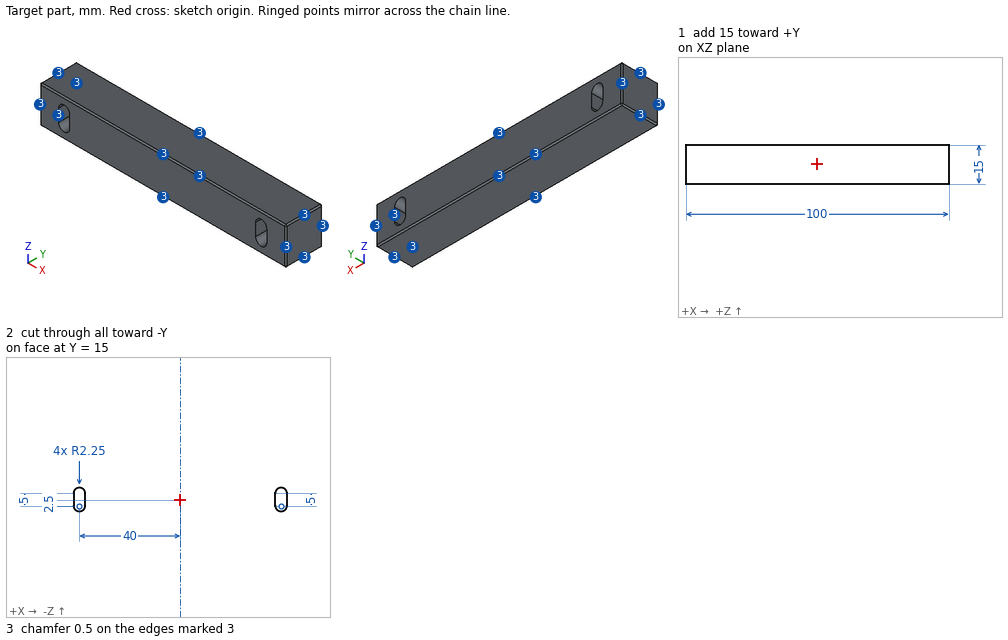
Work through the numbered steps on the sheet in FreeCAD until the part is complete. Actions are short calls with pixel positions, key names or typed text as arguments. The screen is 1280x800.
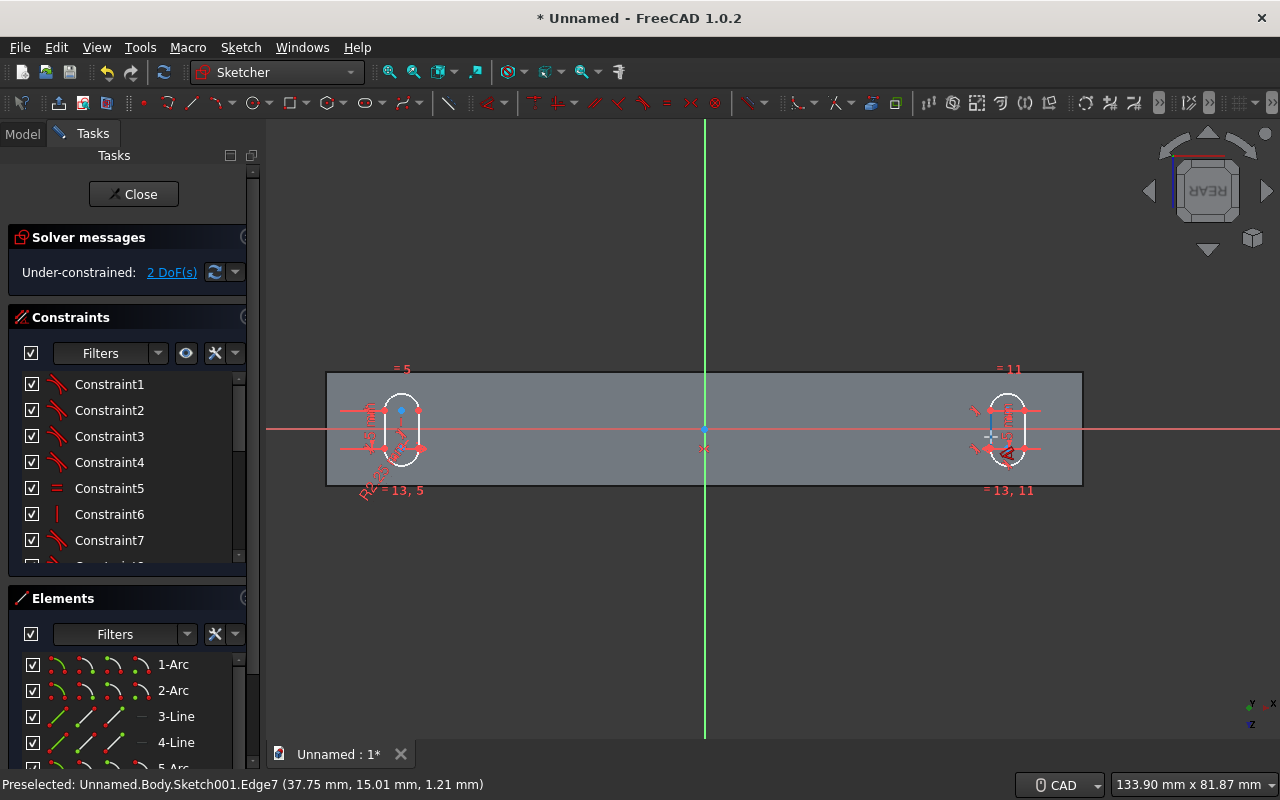
click(402, 449)
click(553, 483)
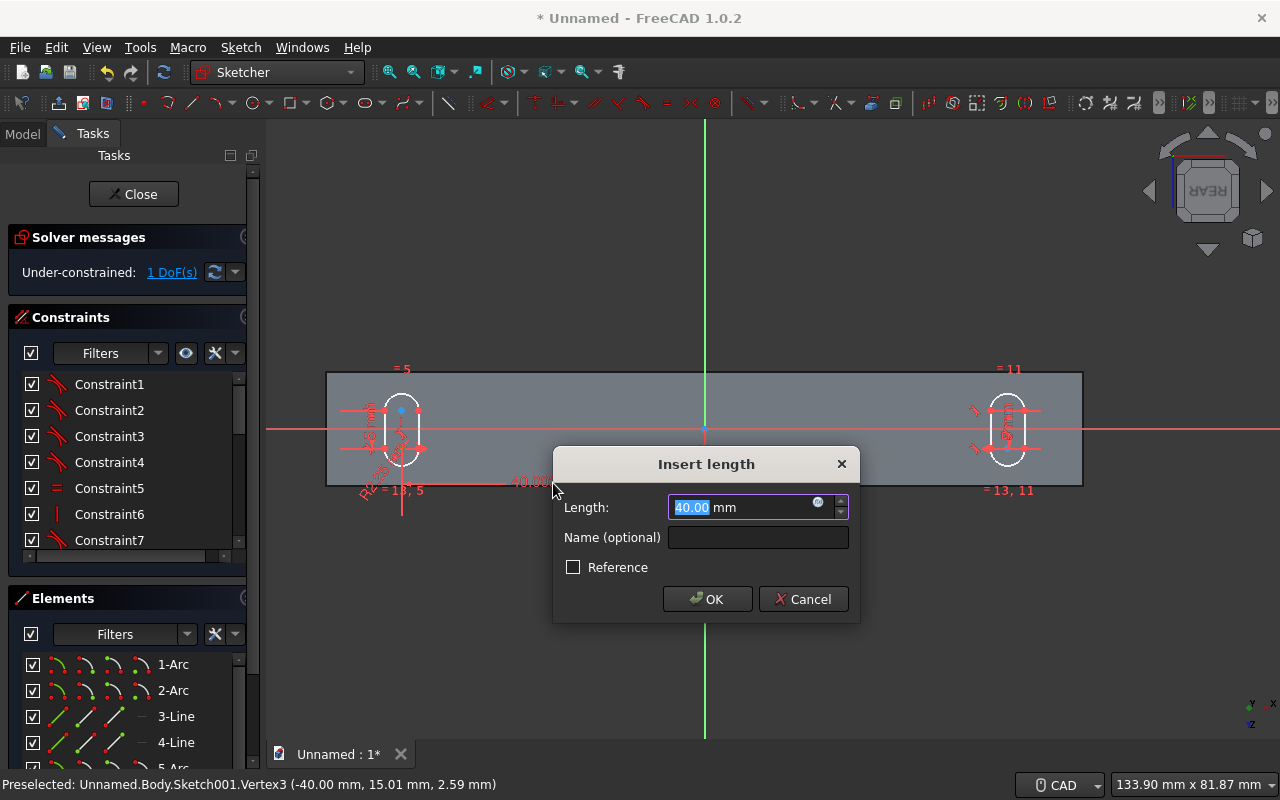
text(40)
key(Return)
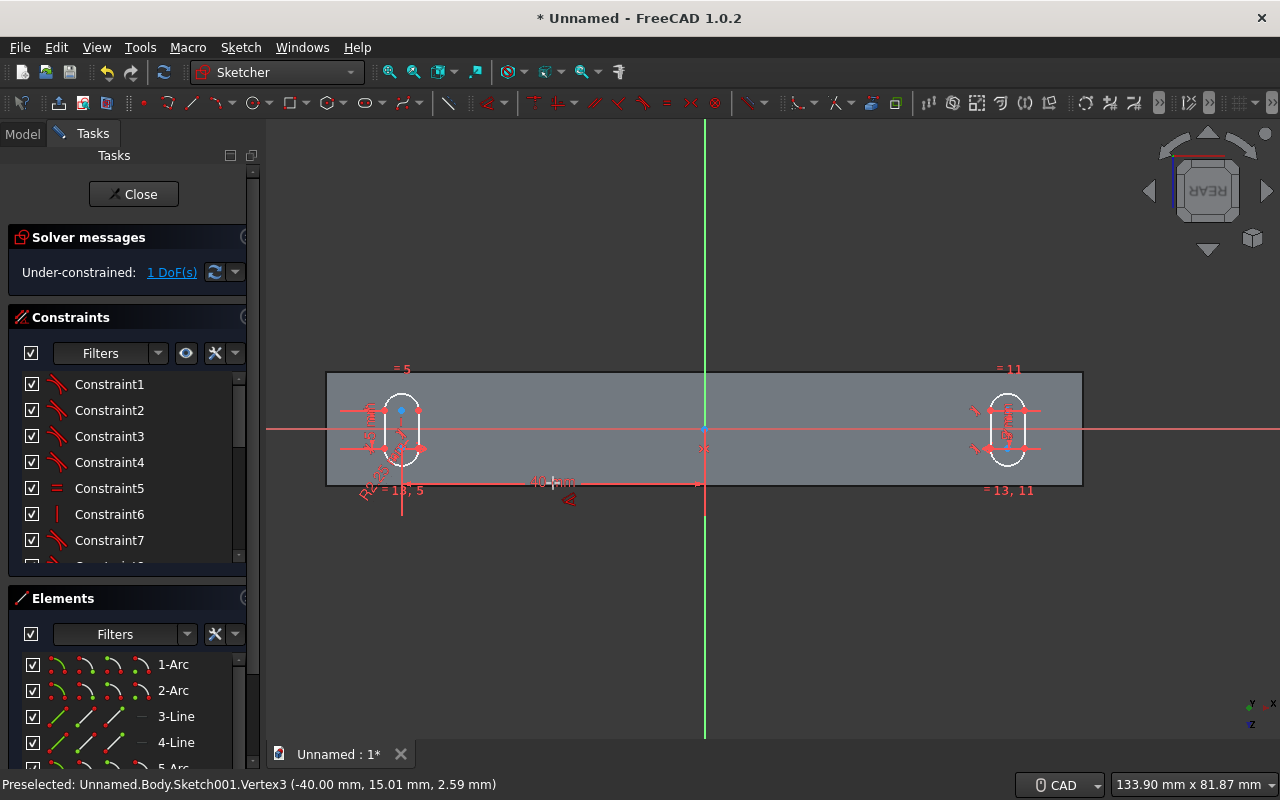
scroll(385, 449, up, 4)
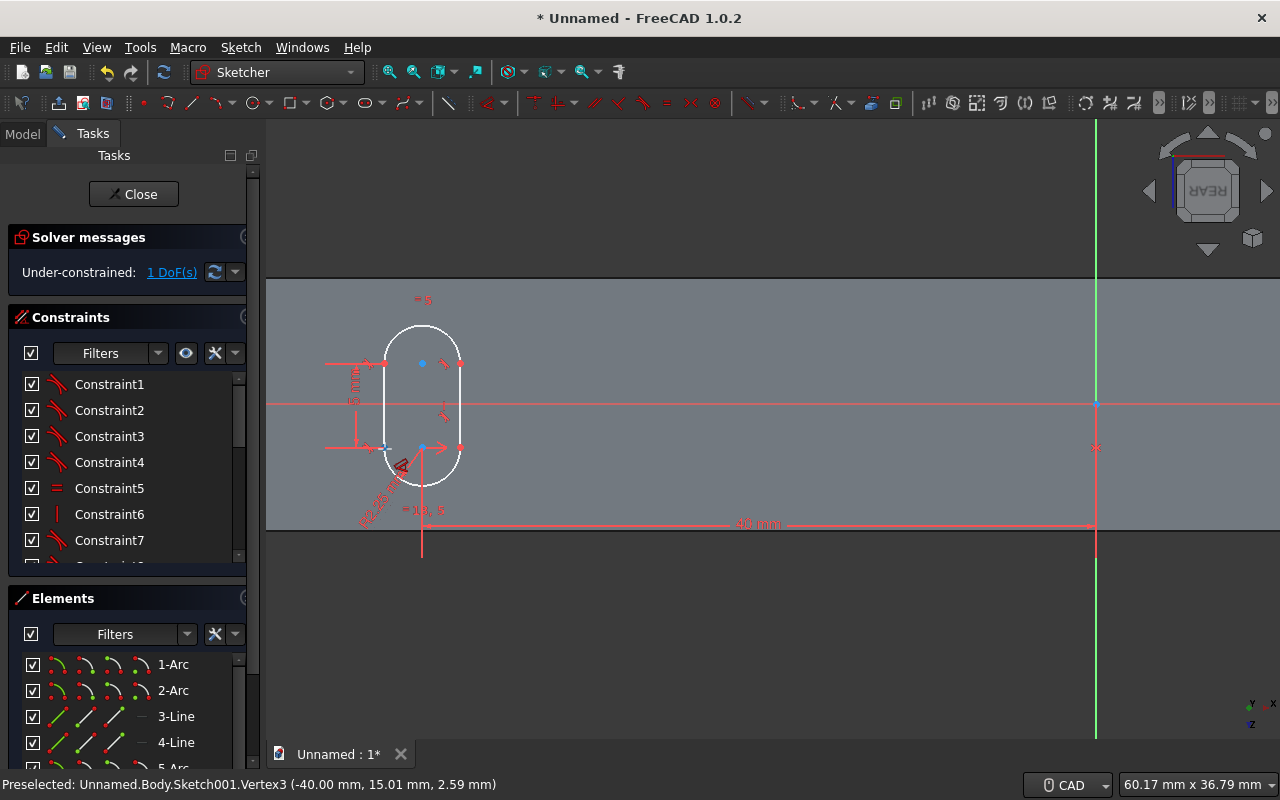
click(384, 448)
click(350, 426)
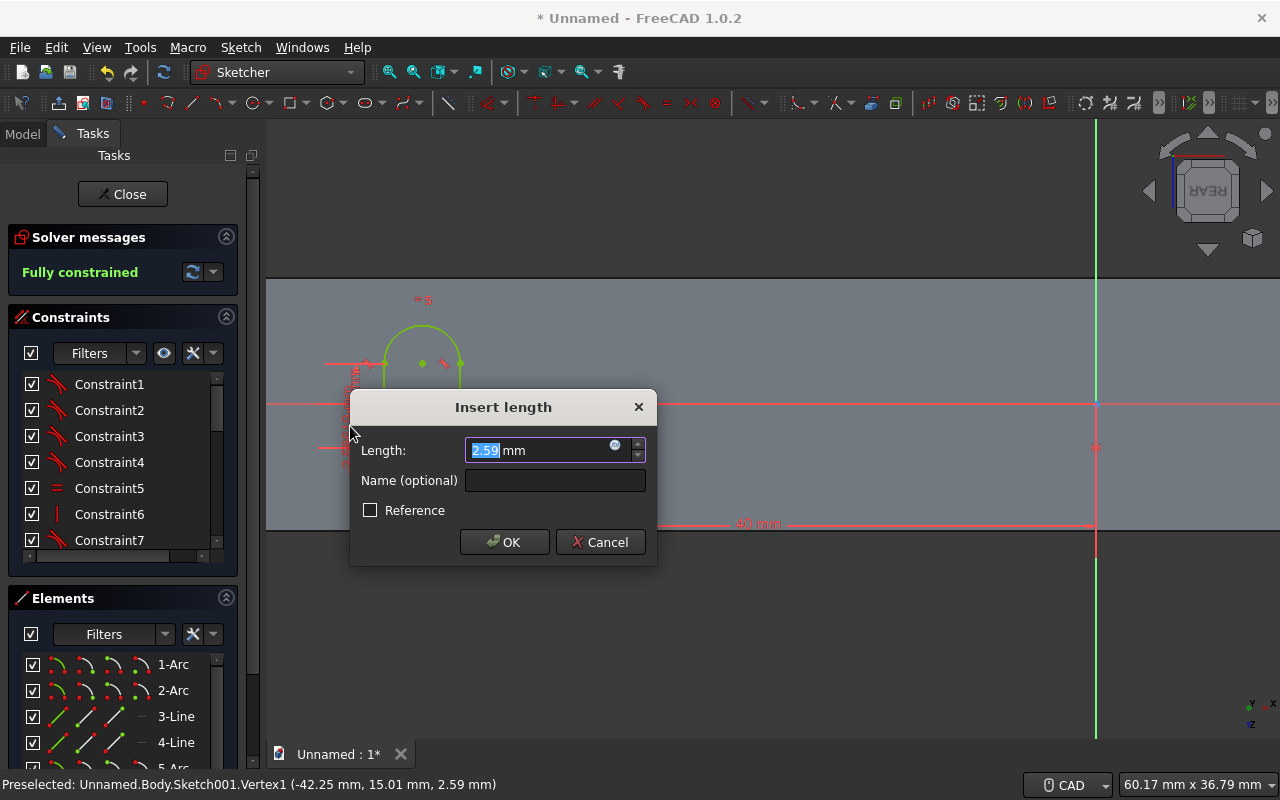
text(2.5)
key(Return)
key(Escape)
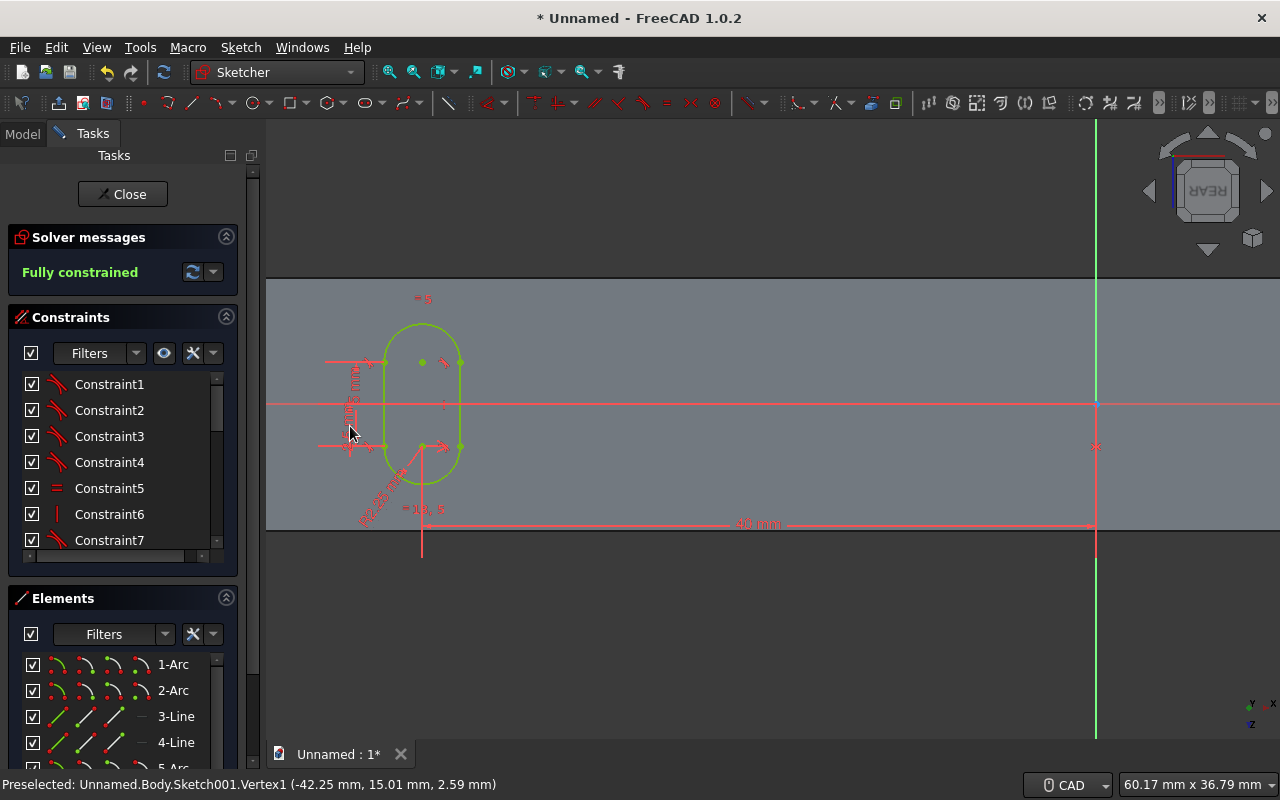
click(123, 194)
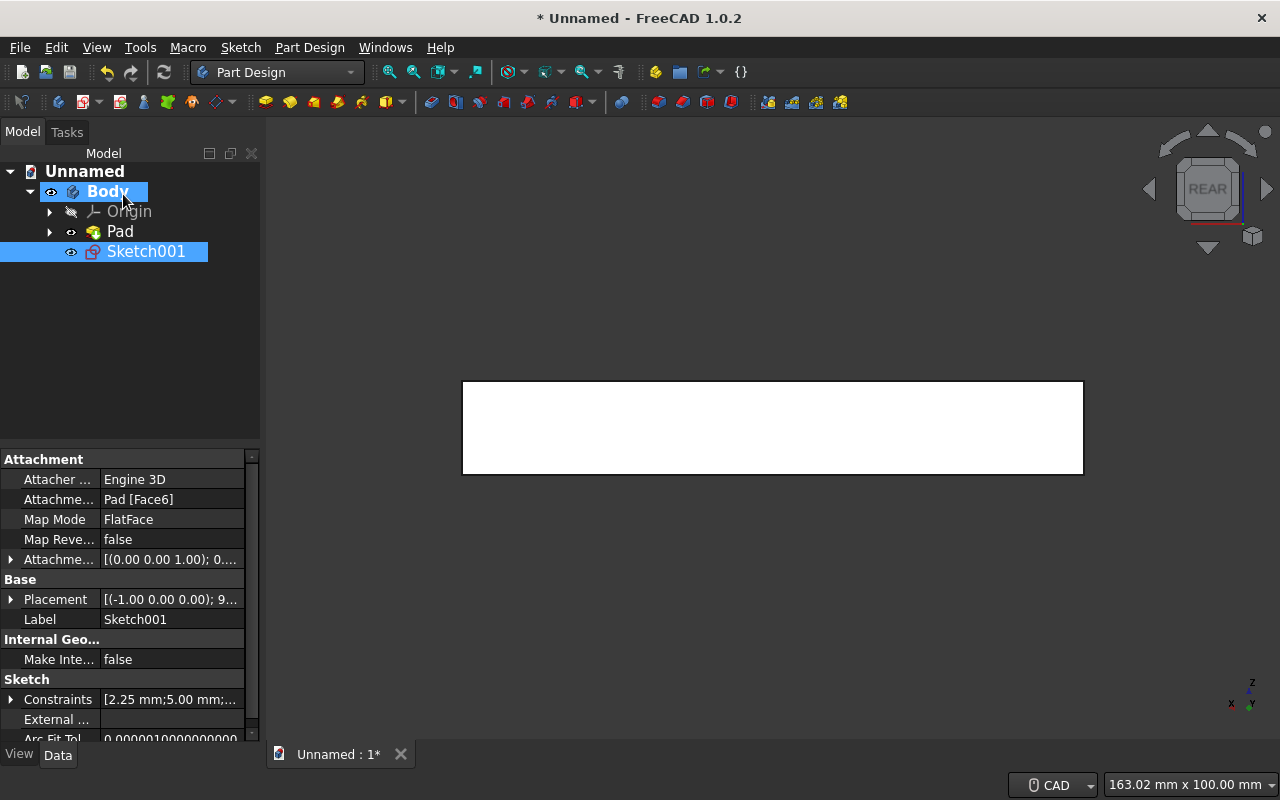
click(432, 102)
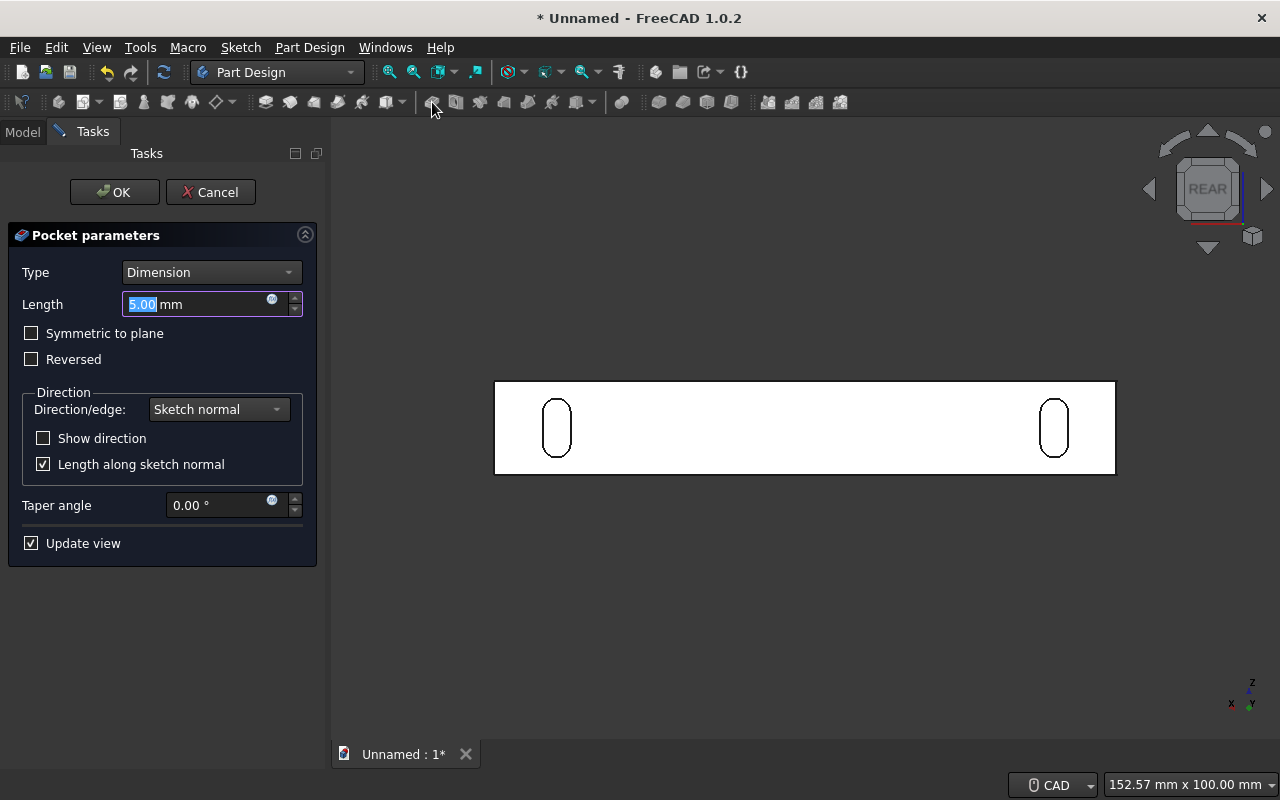
click(212, 272)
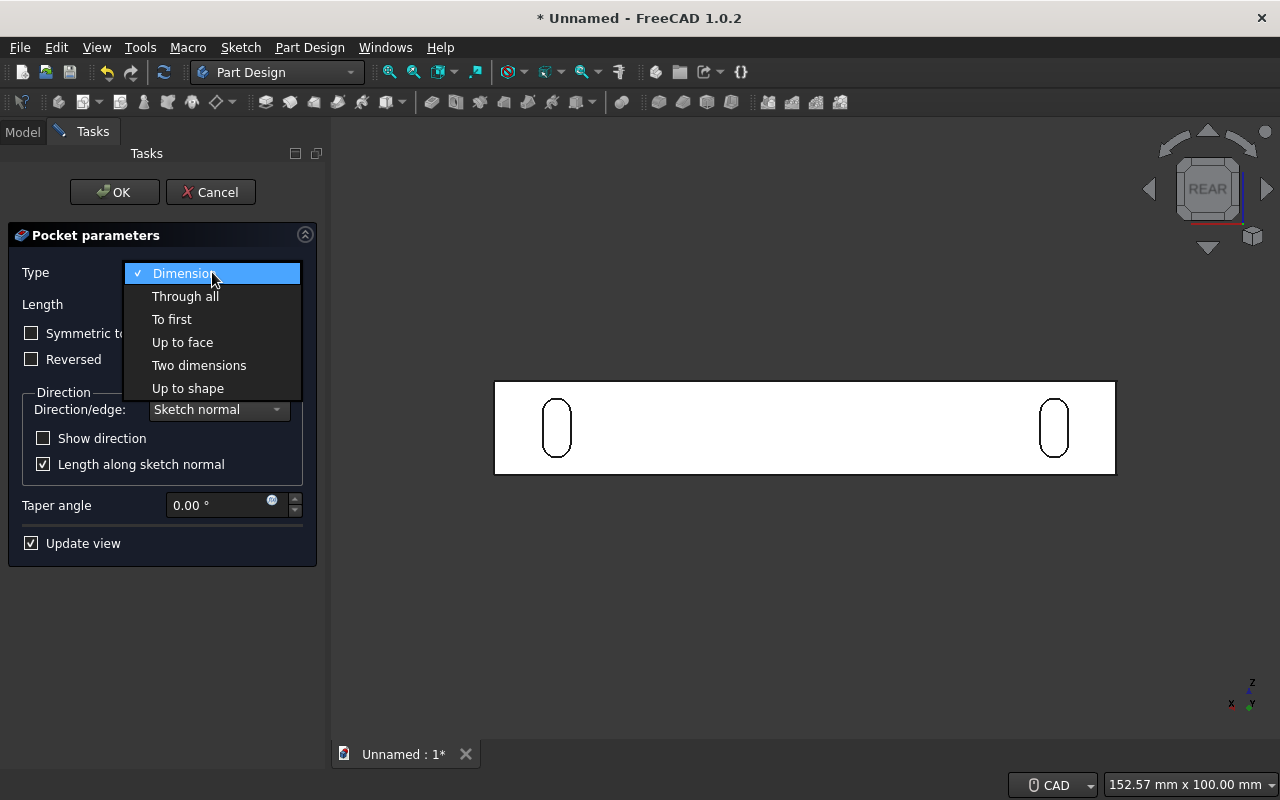
click(212, 296)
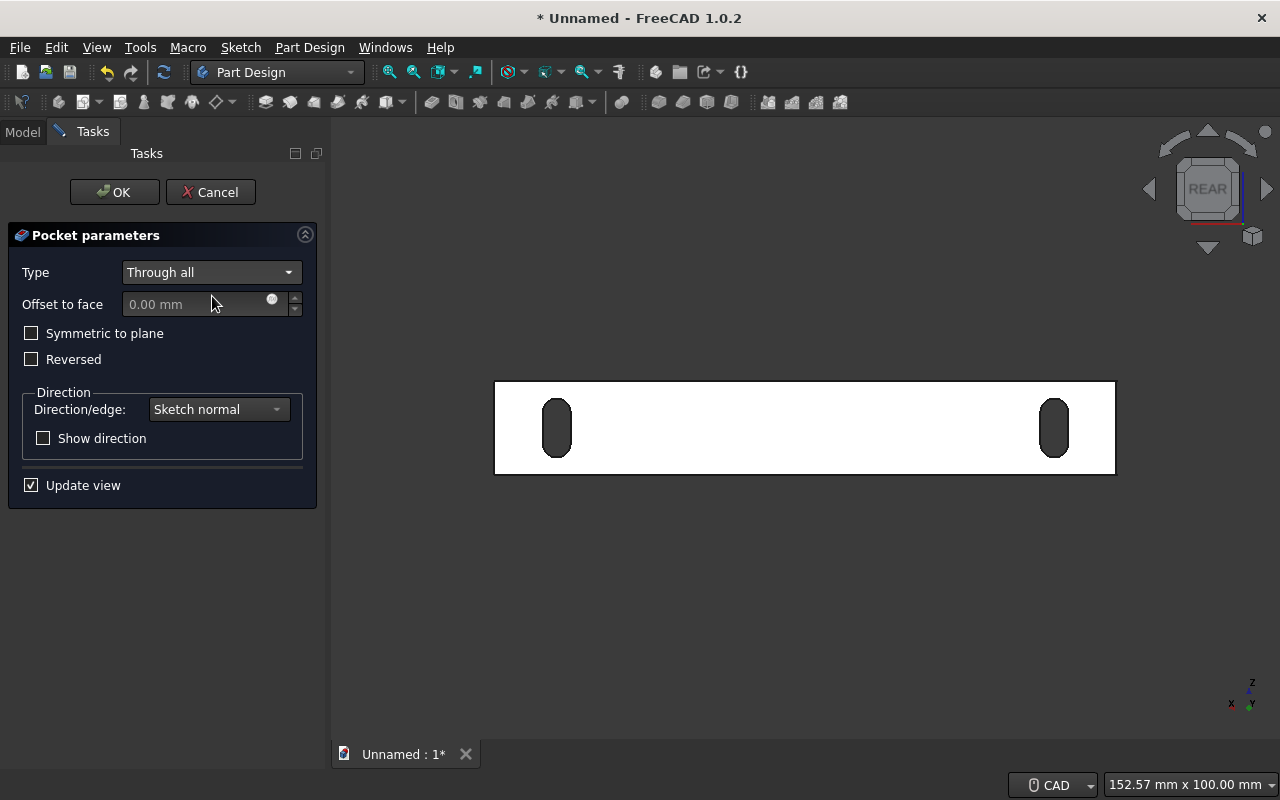
click(115, 192)